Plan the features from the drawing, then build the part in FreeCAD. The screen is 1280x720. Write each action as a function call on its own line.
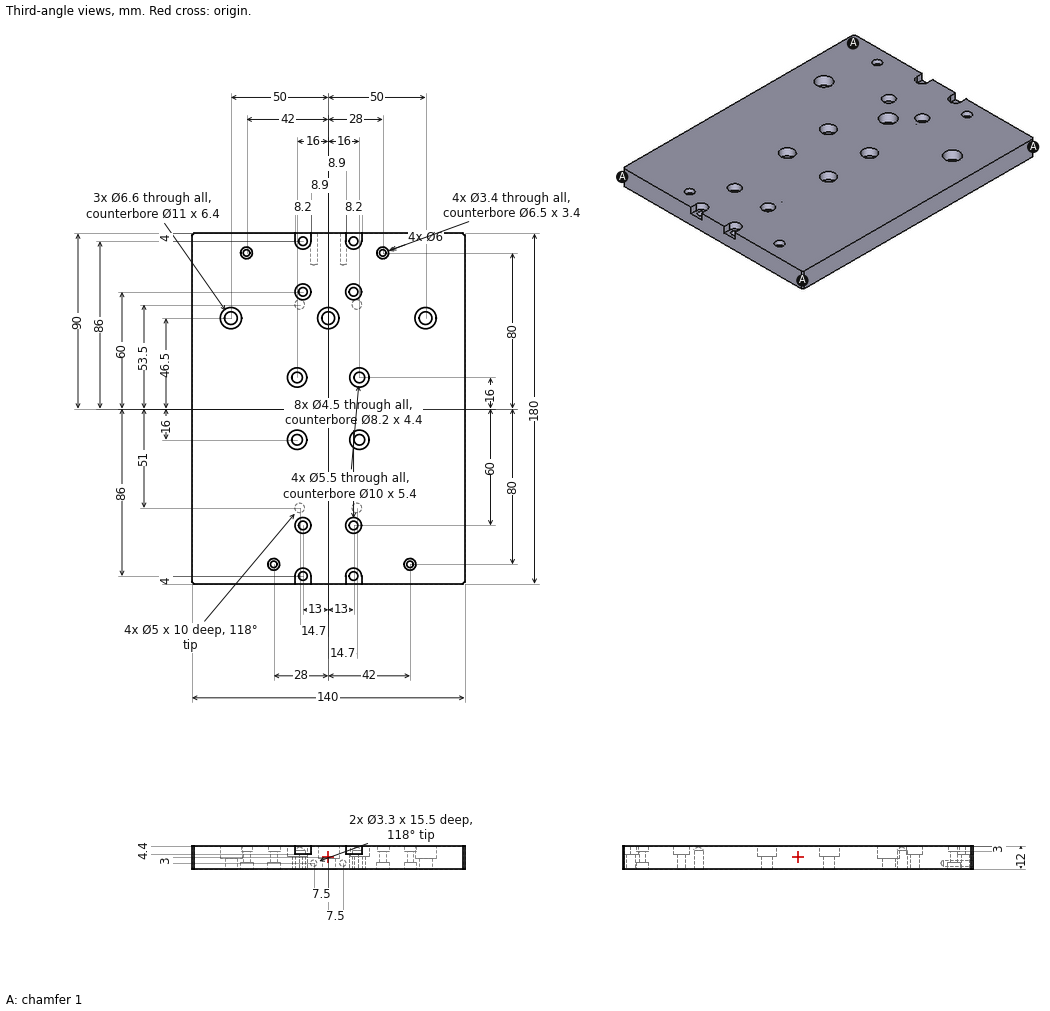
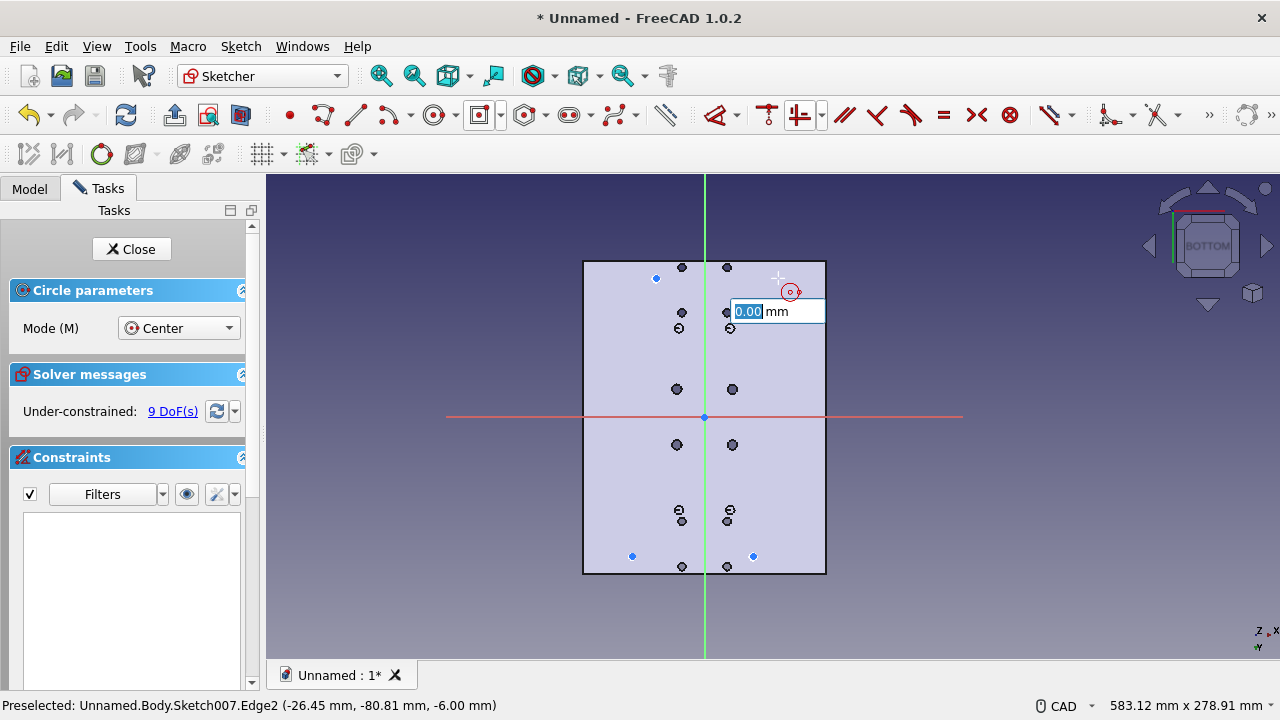
scroll(780, 276, up, 9)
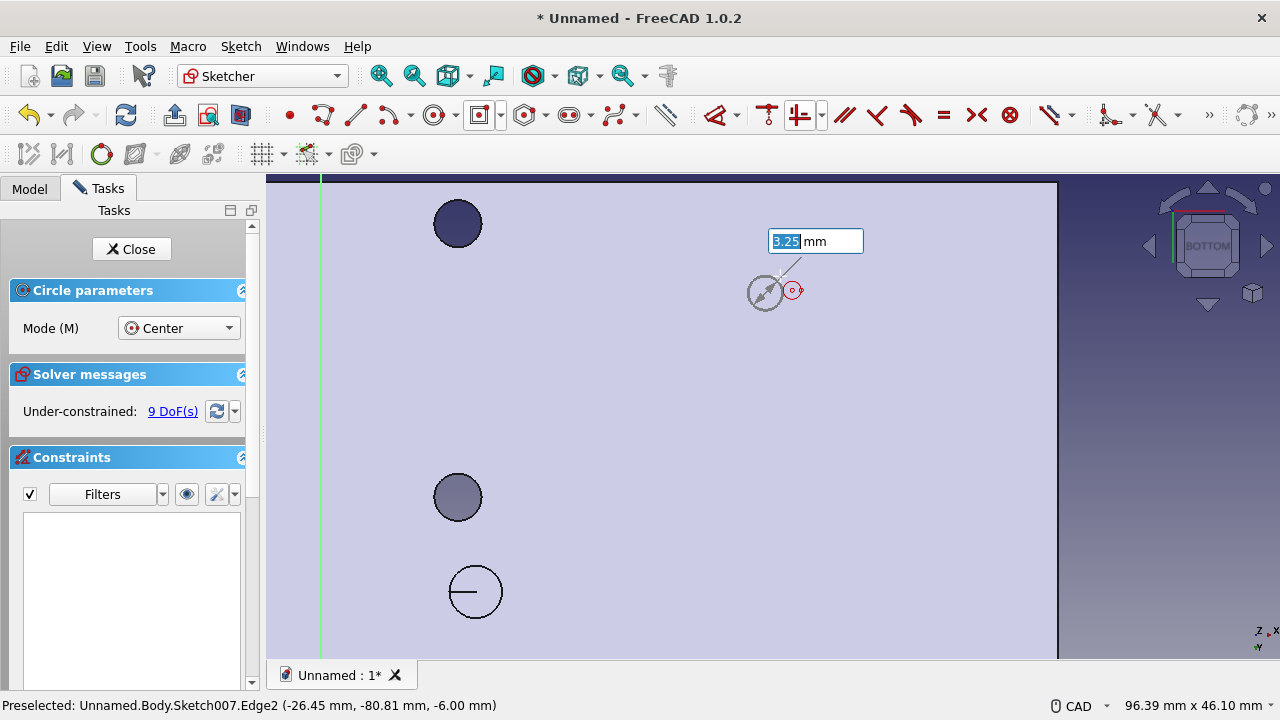
click(776, 274)
key(Escape)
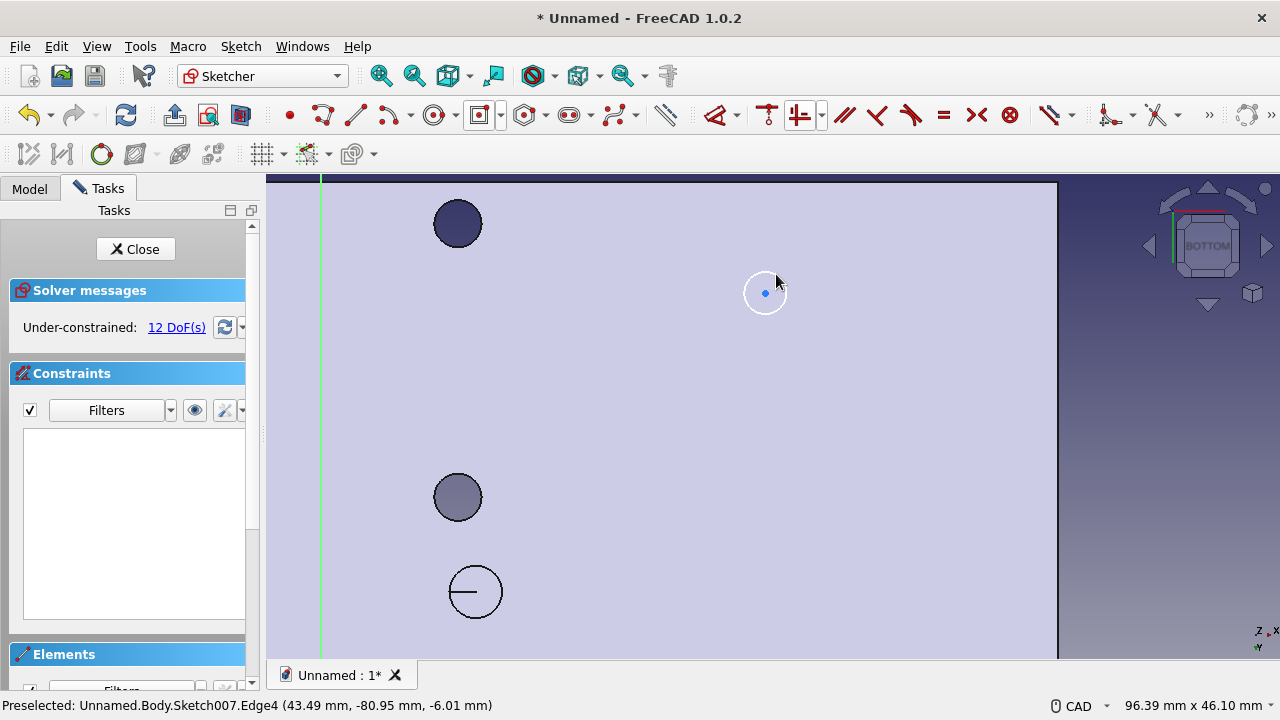
scroll(780, 276, down, 9)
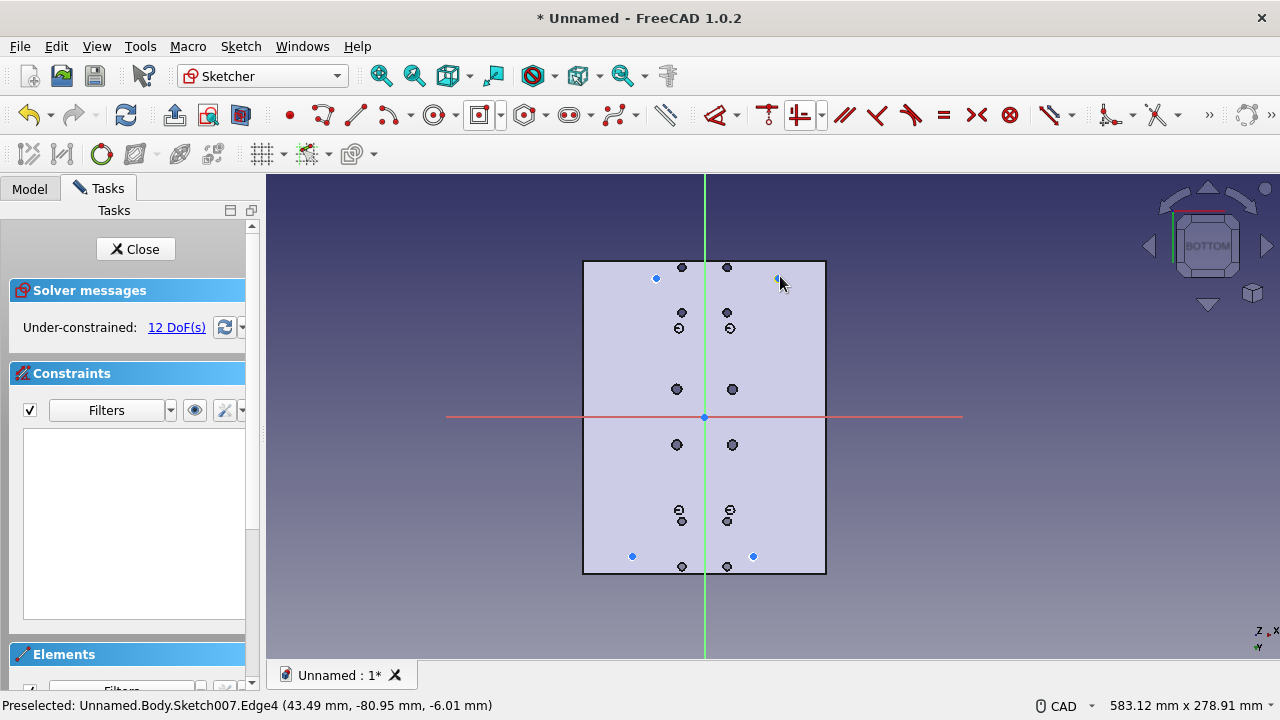
scroll(756, 554, up, 7)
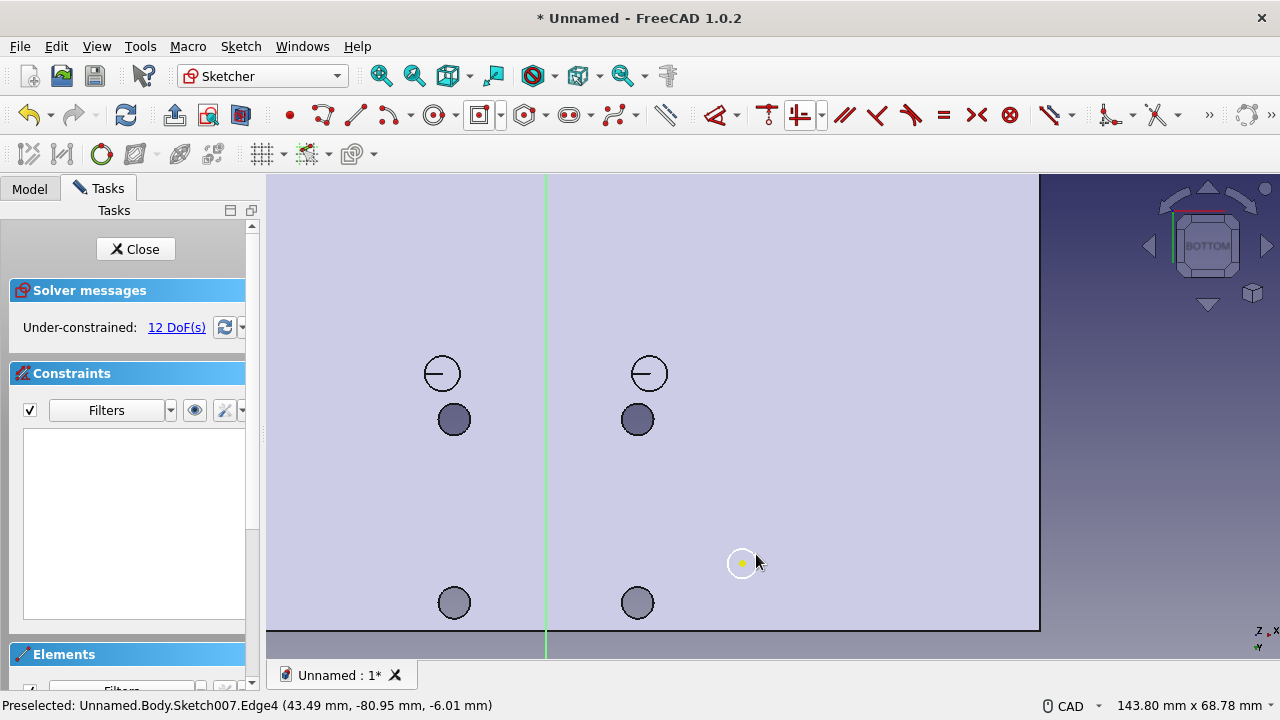
click(753, 553)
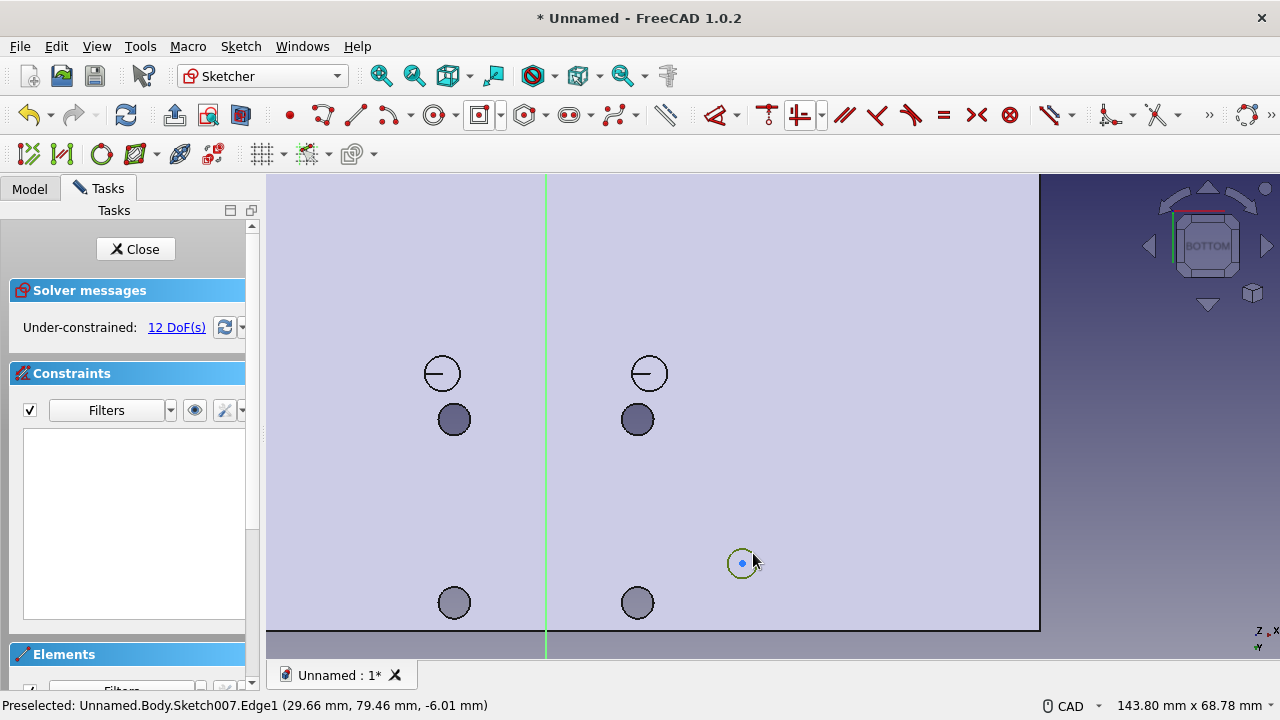
scroll(756, 554, down, 7)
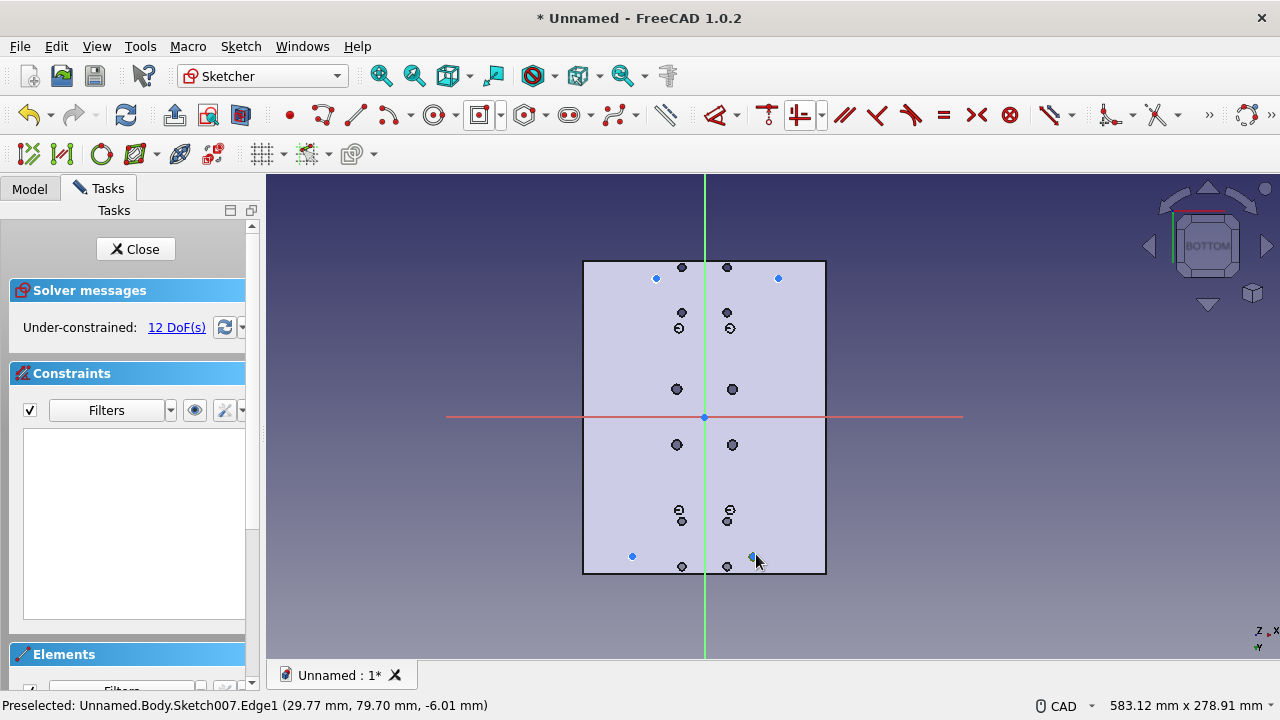
scroll(634, 555, up, 8)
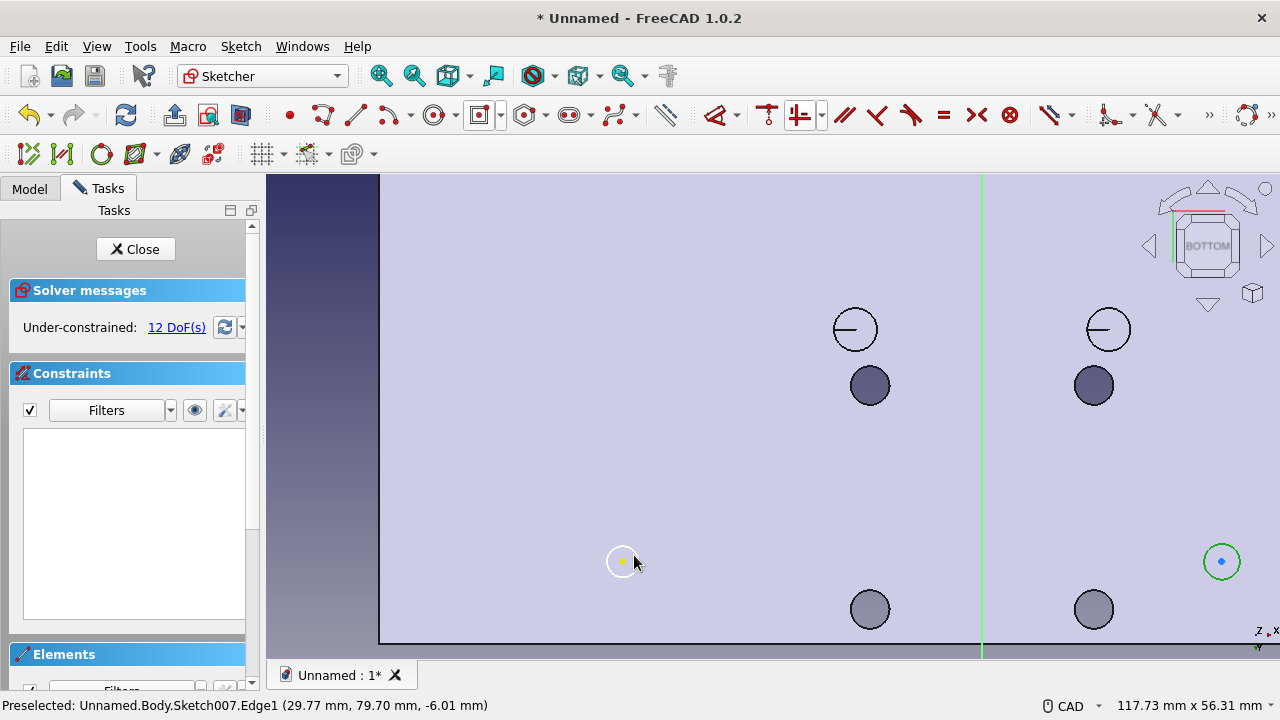
click(634, 551)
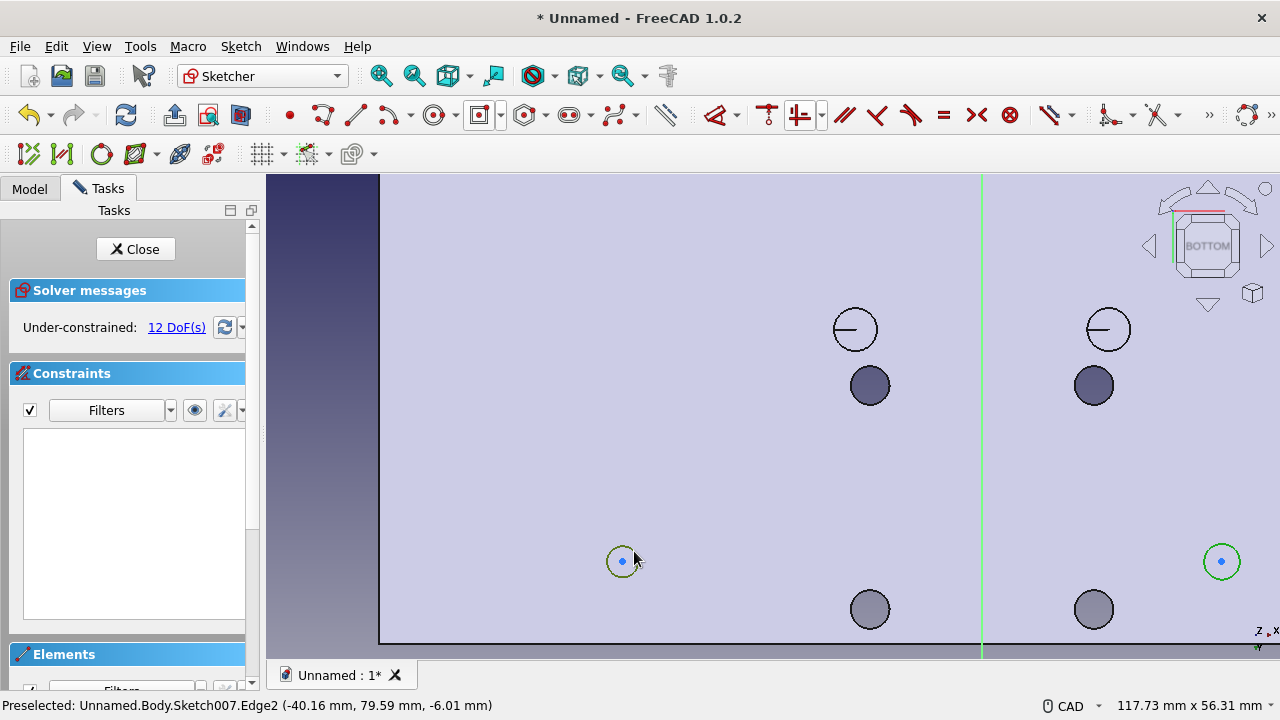
scroll(634, 555, down, 8)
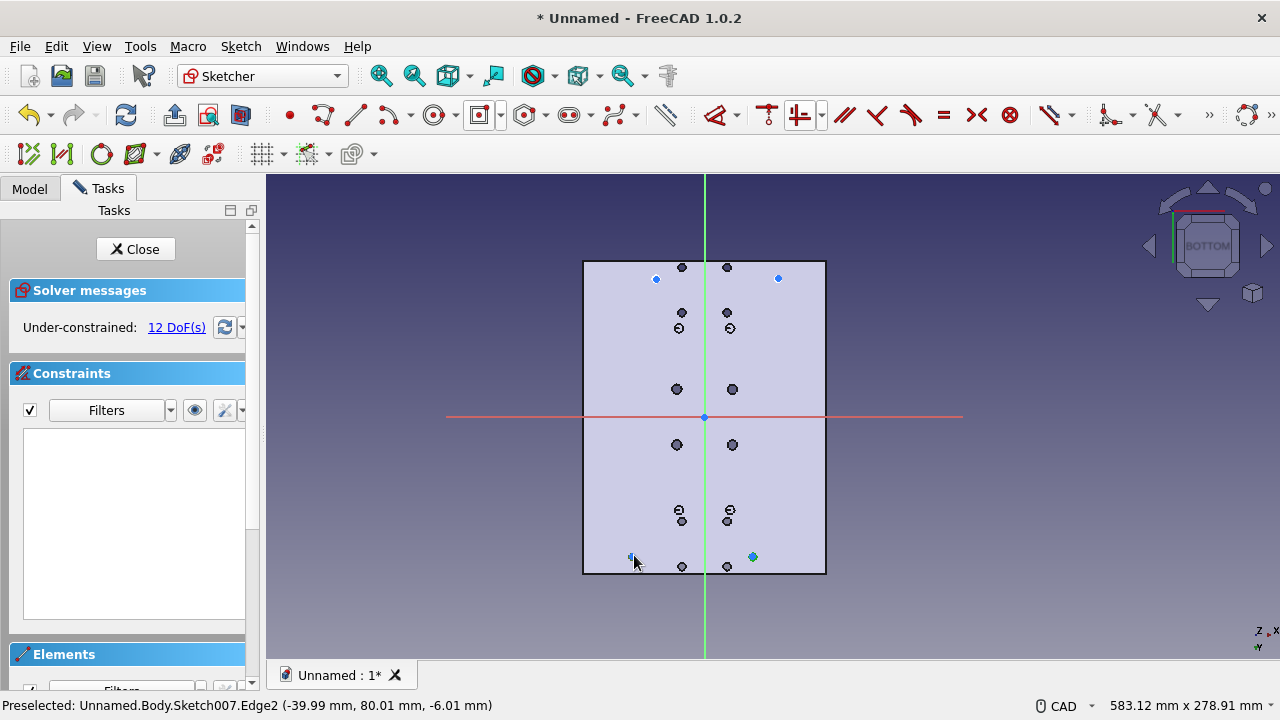
scroll(659, 276, up, 7)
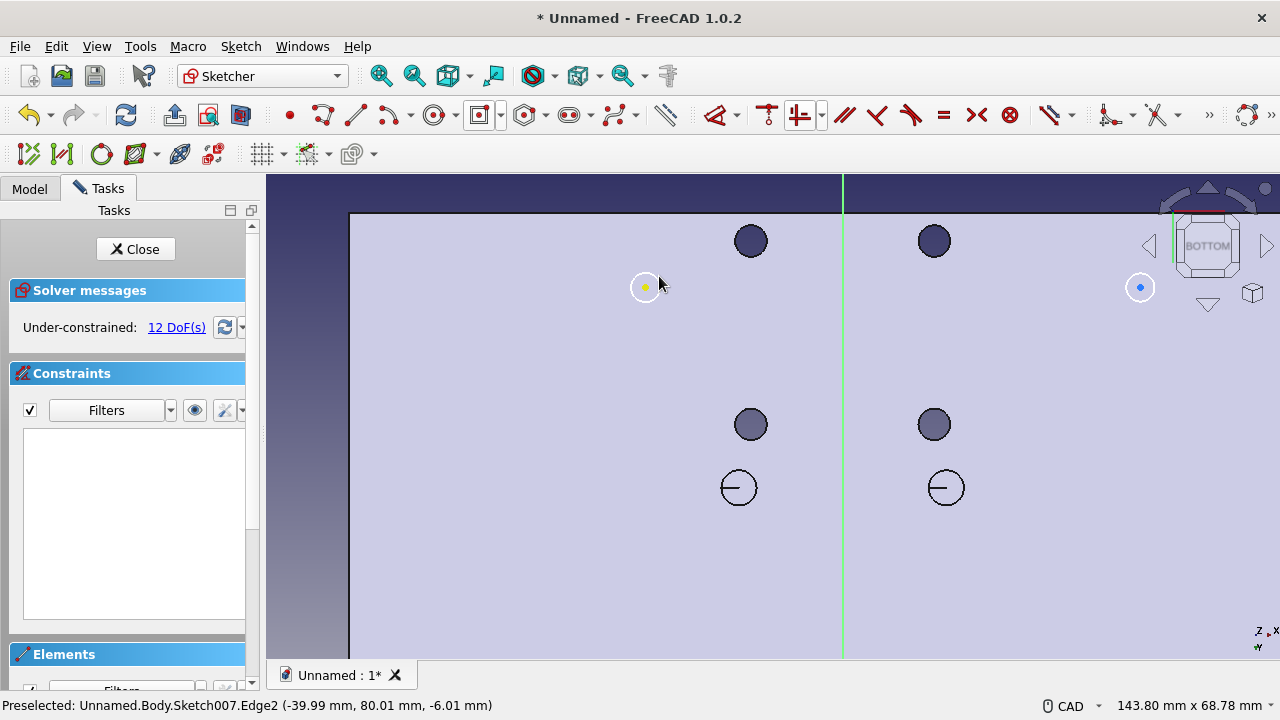
click(656, 277)